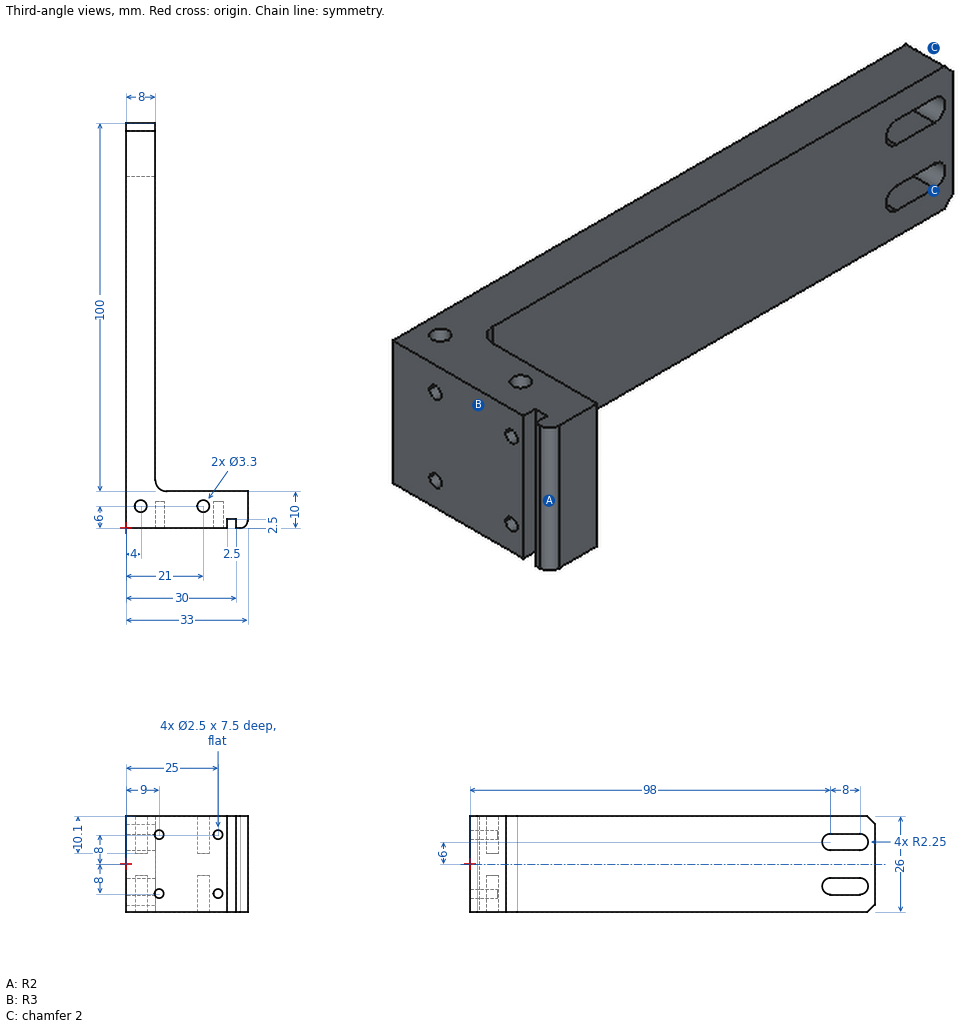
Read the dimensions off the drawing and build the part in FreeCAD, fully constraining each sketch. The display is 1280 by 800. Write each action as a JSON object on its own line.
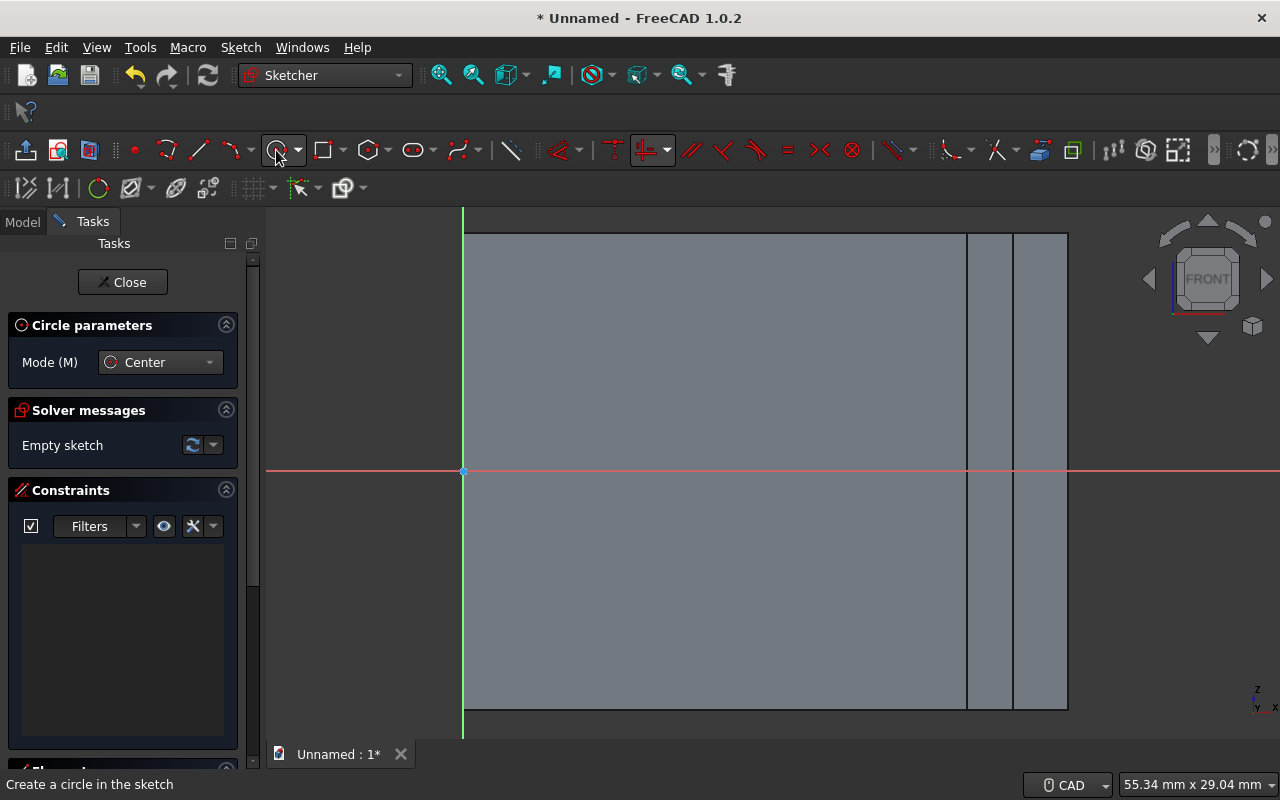
{"action": "left_click", "coordinate": [921, 325]}
{"action": "mouse_move", "coordinate": [937, 309]}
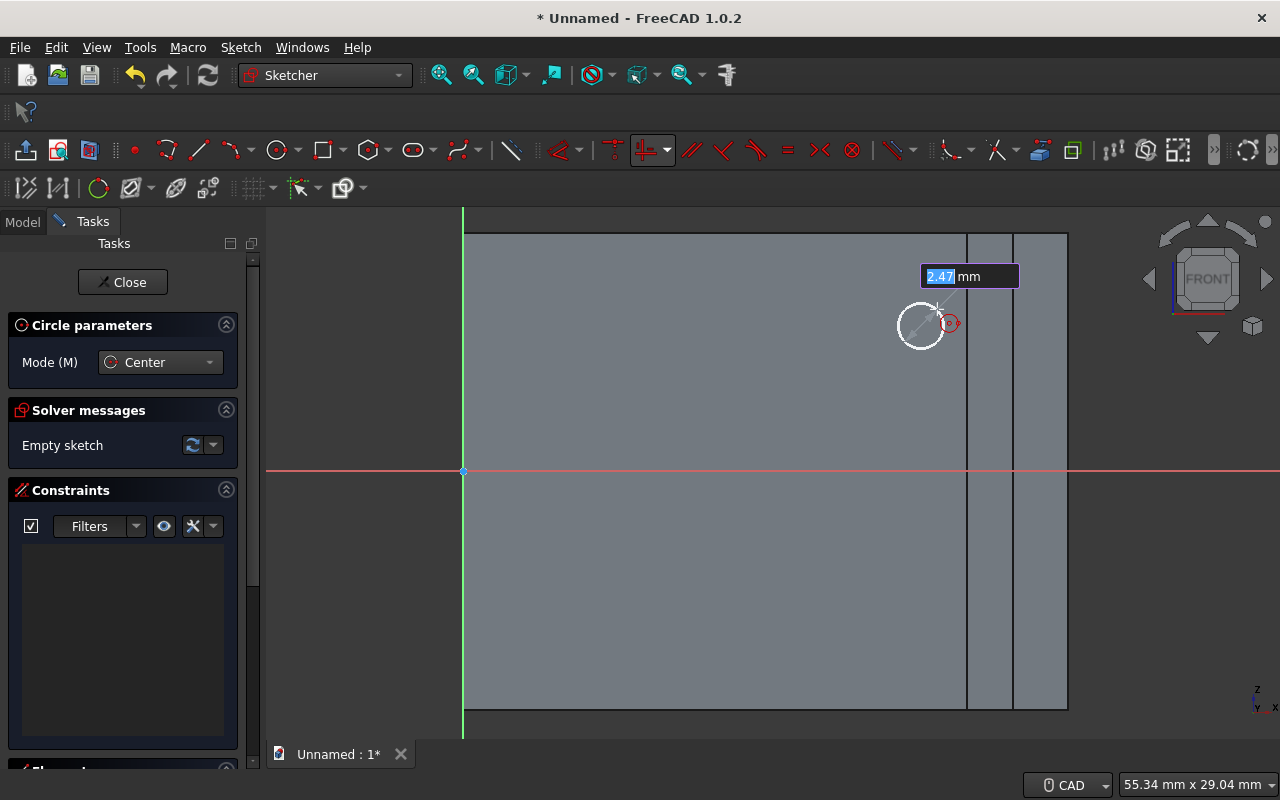
{"action": "type", "text": "2.5"}
{"action": "key", "text": "Return"}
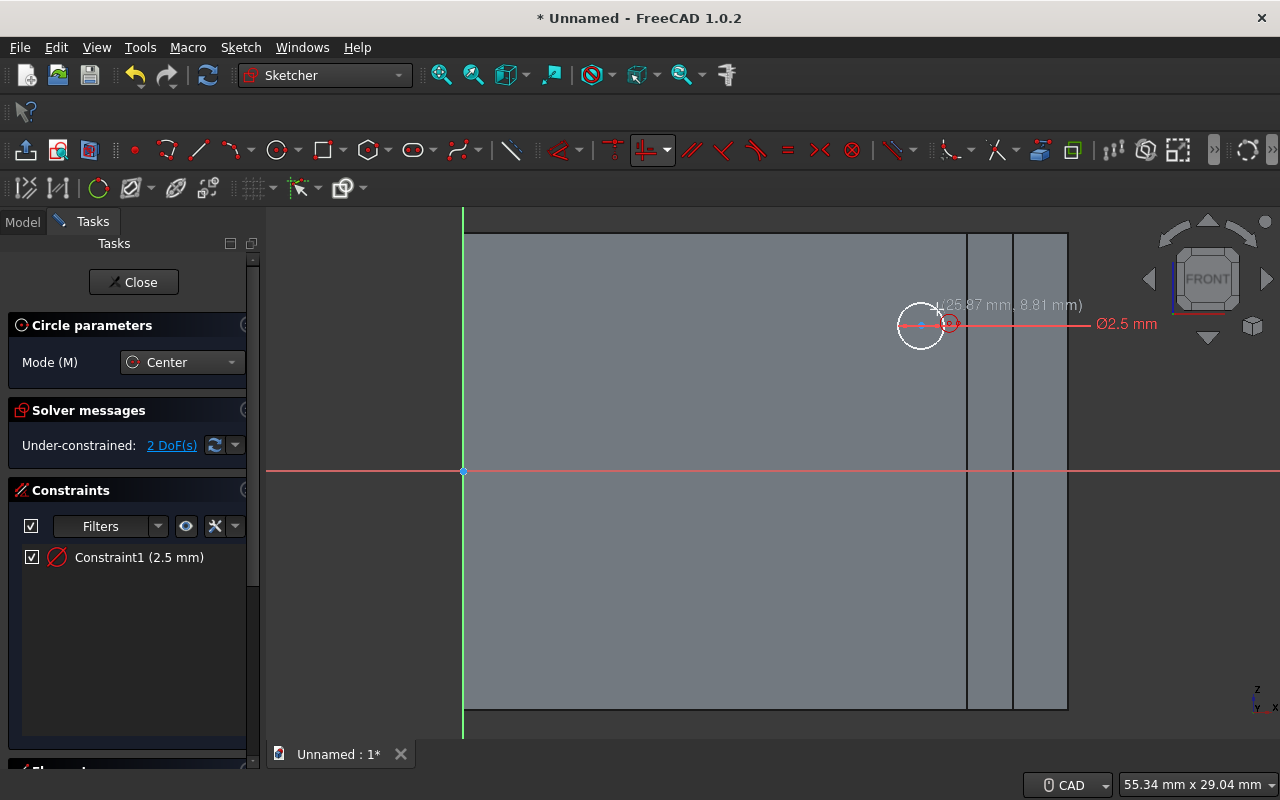
{"action": "left_click", "coordinate": [628, 325]}
{"action": "mouse_move", "coordinate": [644, 309]}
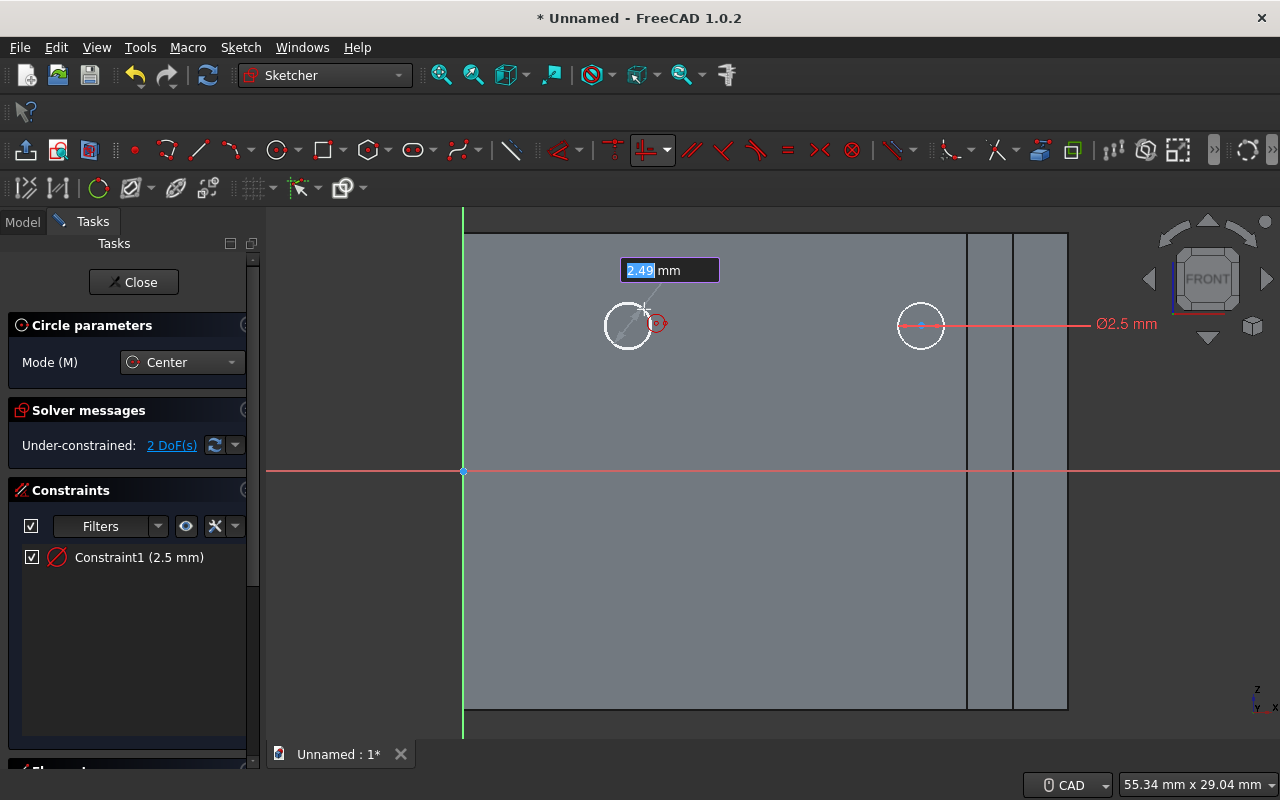
{"action": "type", "text": "2.5"}
{"action": "key", "text": "Return"}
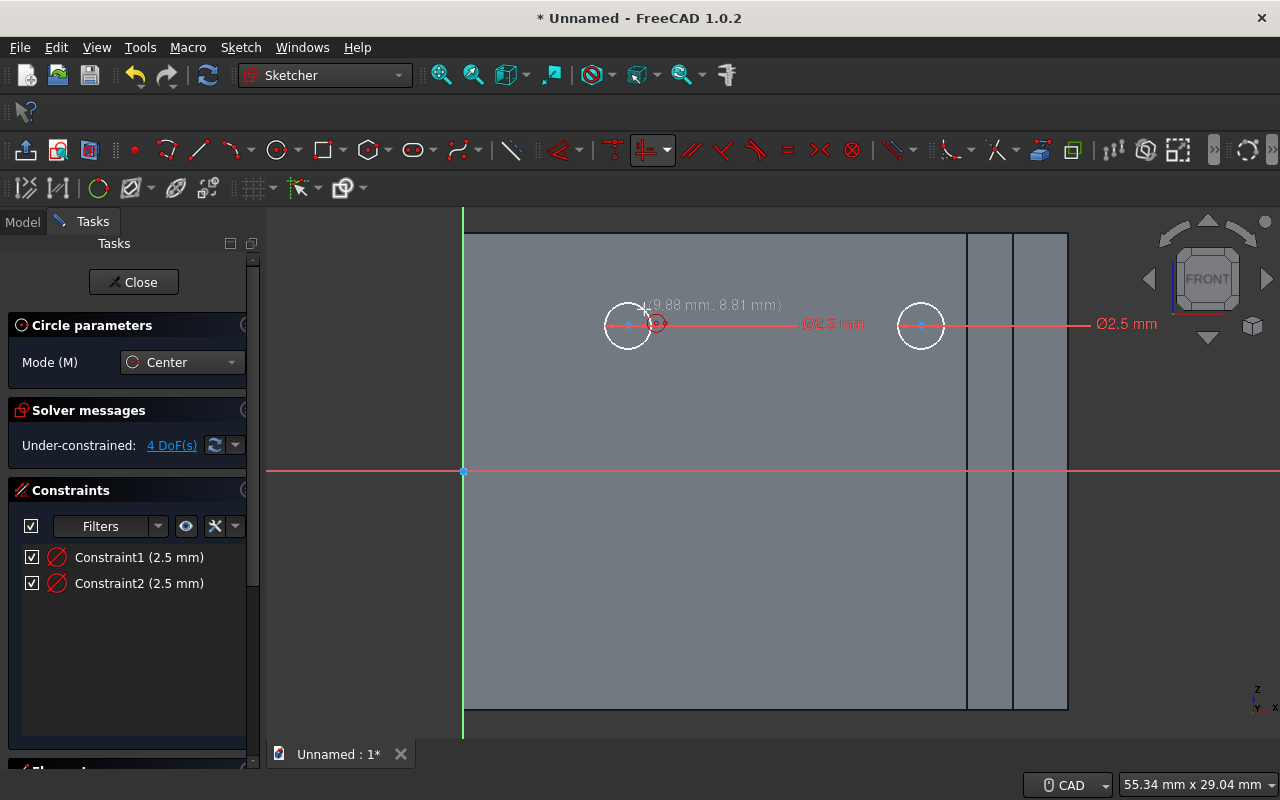
{"action": "left_click", "coordinate": [628, 618]}
{"action": "mouse_move", "coordinate": [644, 602]}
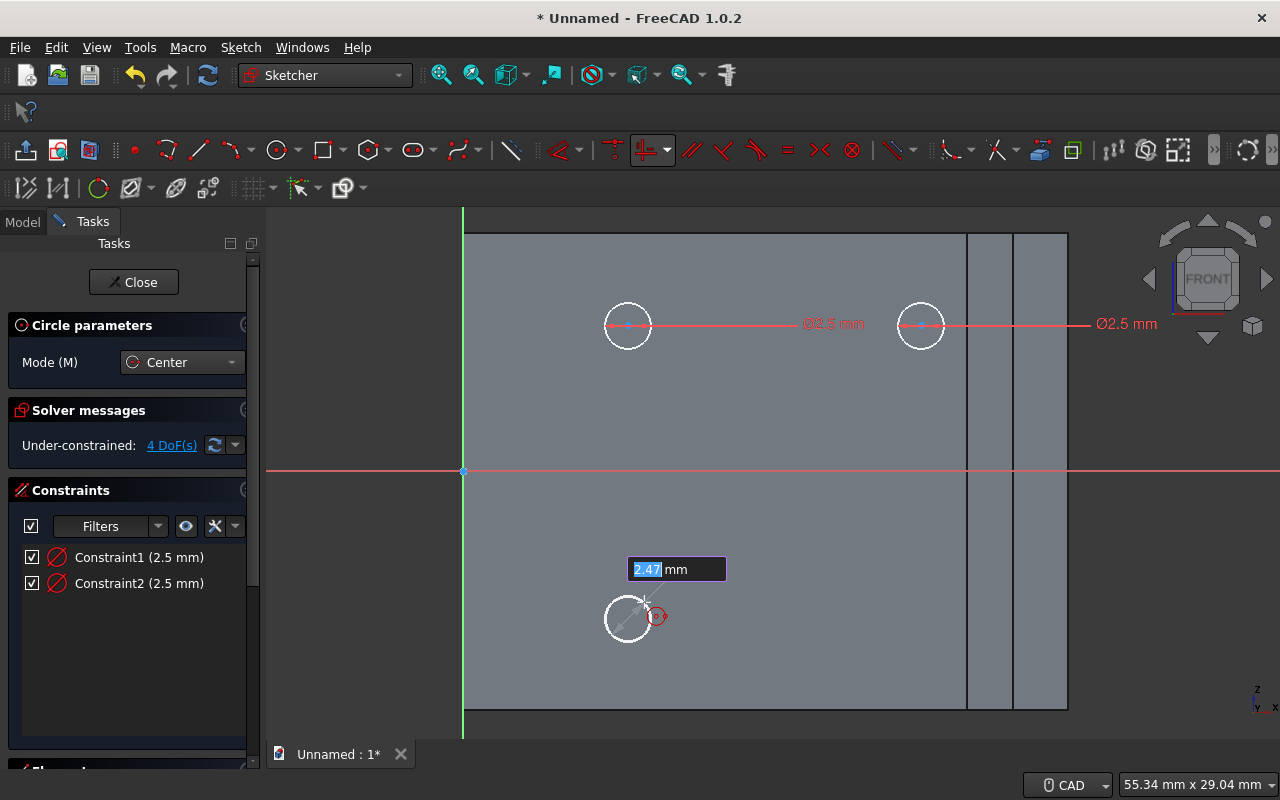
{"action": "type", "text": "2.5"}
{"action": "key", "text": "Return"}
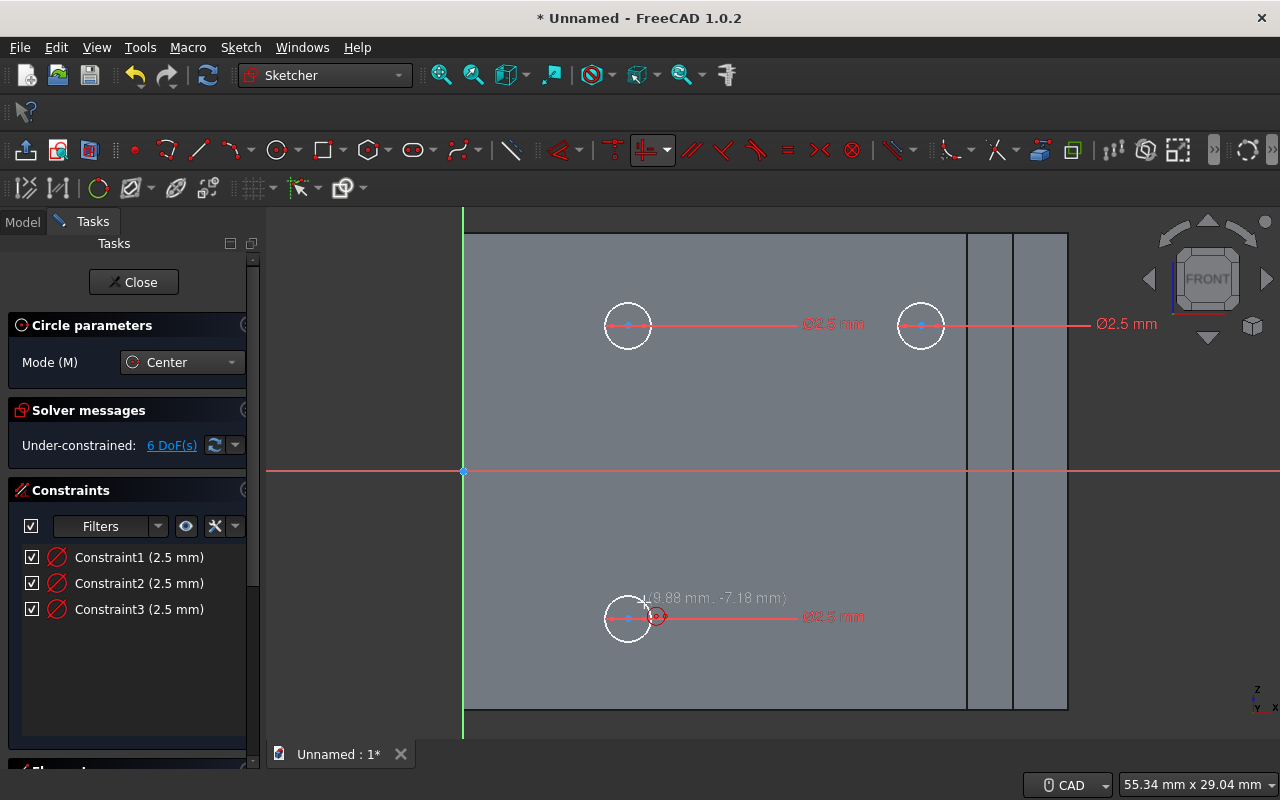
{"action": "left_click", "coordinate": [921, 618]}
{"action": "mouse_move", "coordinate": [937, 602]}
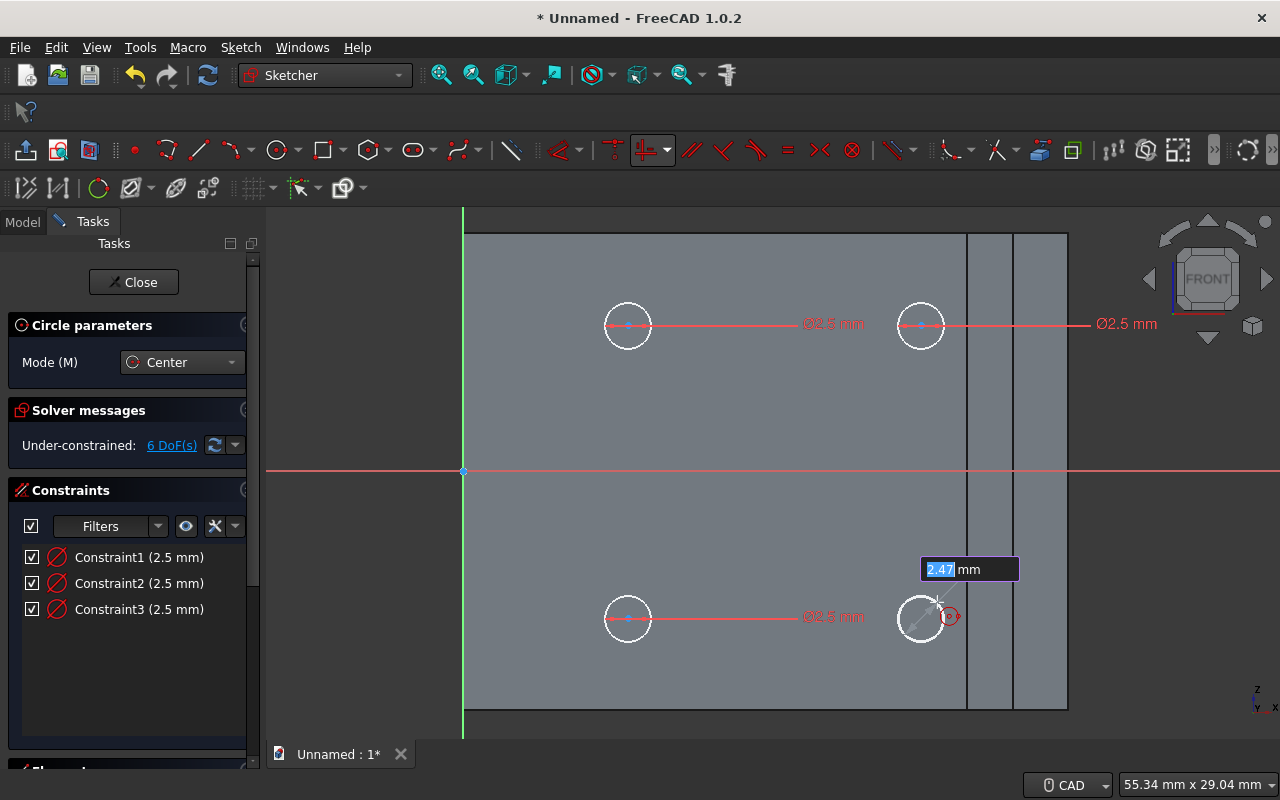
{"action": "type", "text": "2.5"}
{"action": "key", "text": "Return"}
{"action": "key", "text": "Escape"}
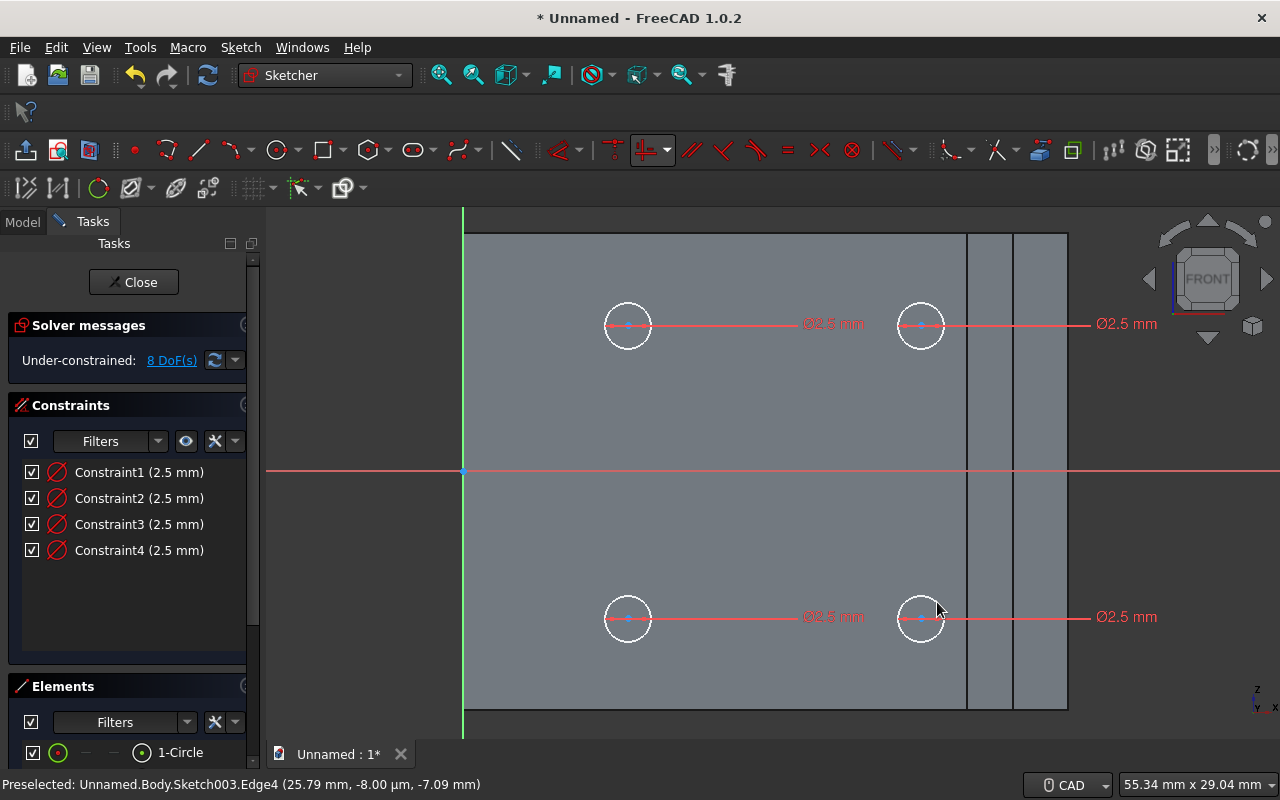
{"action": "left_click", "coordinate": [921, 326]}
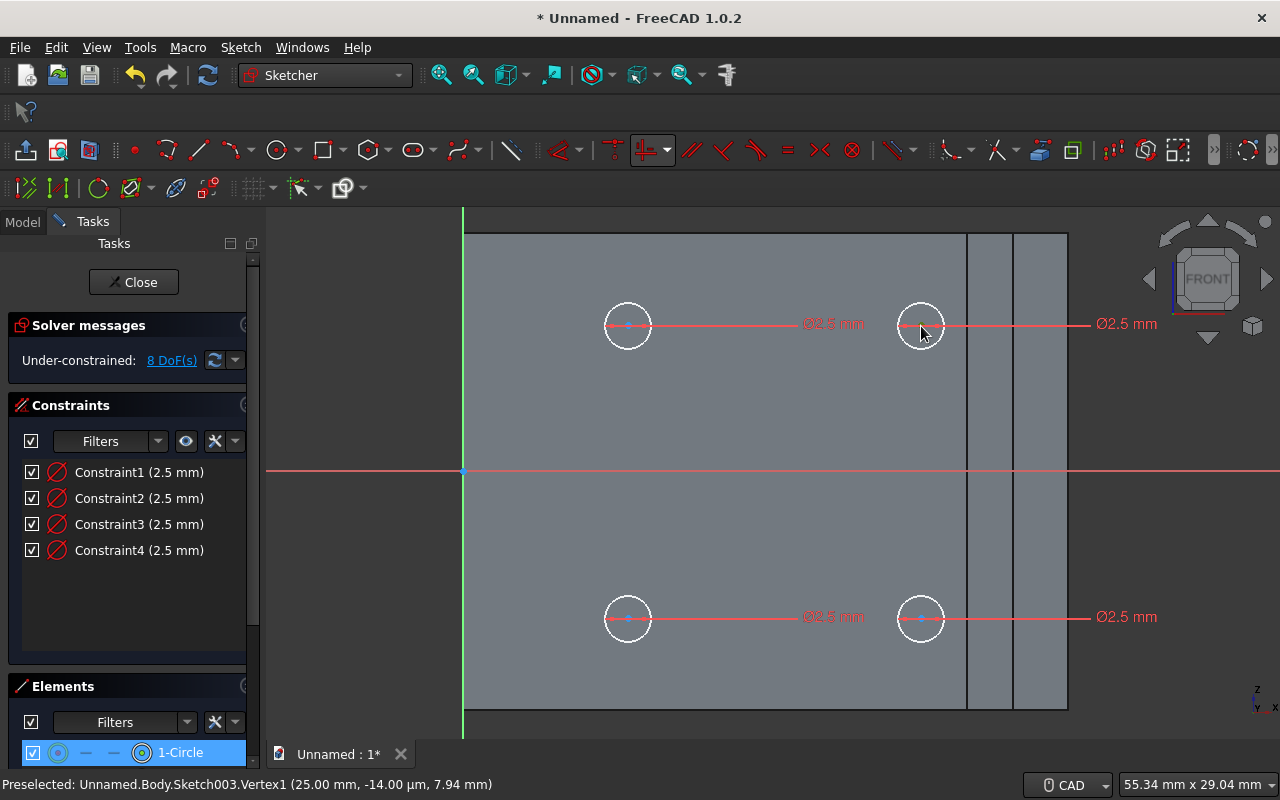
{"action": "left_click", "coordinate": [628, 326]}